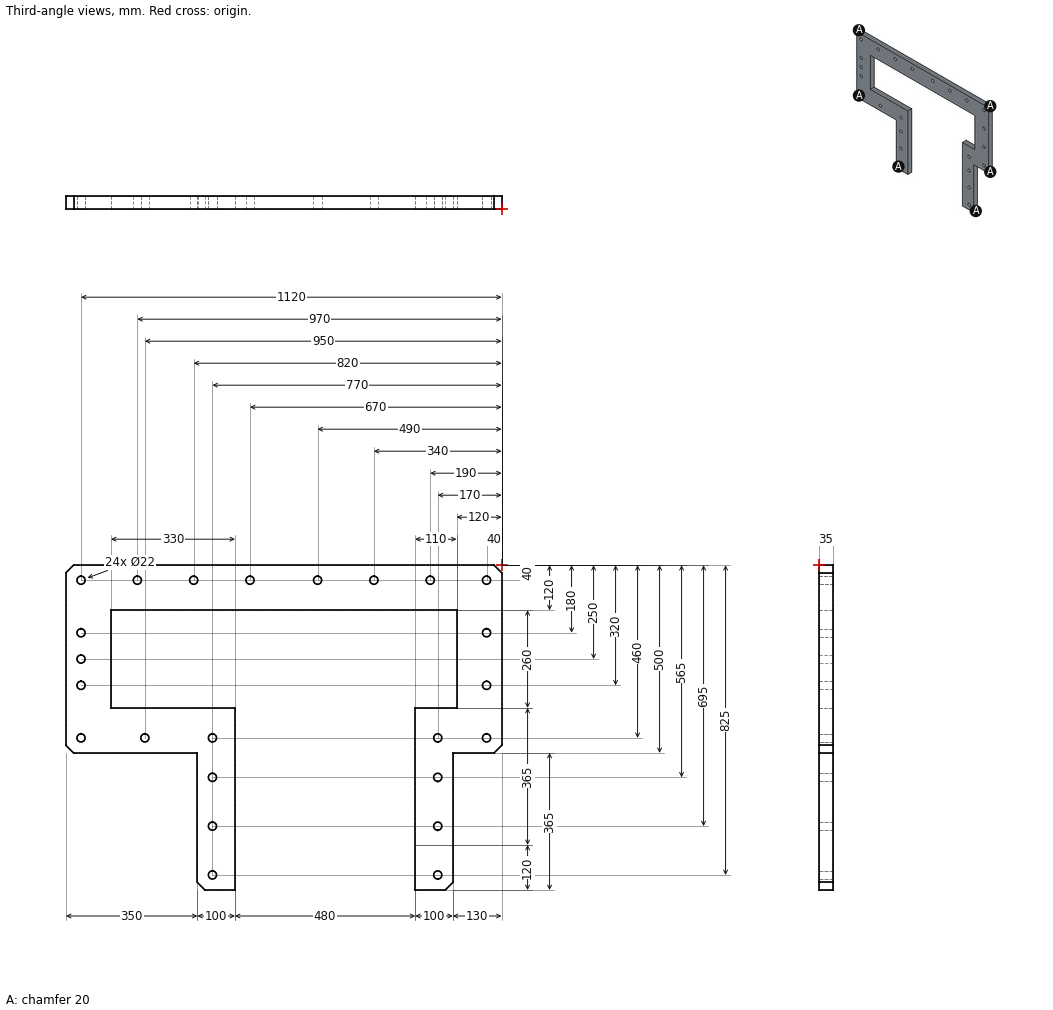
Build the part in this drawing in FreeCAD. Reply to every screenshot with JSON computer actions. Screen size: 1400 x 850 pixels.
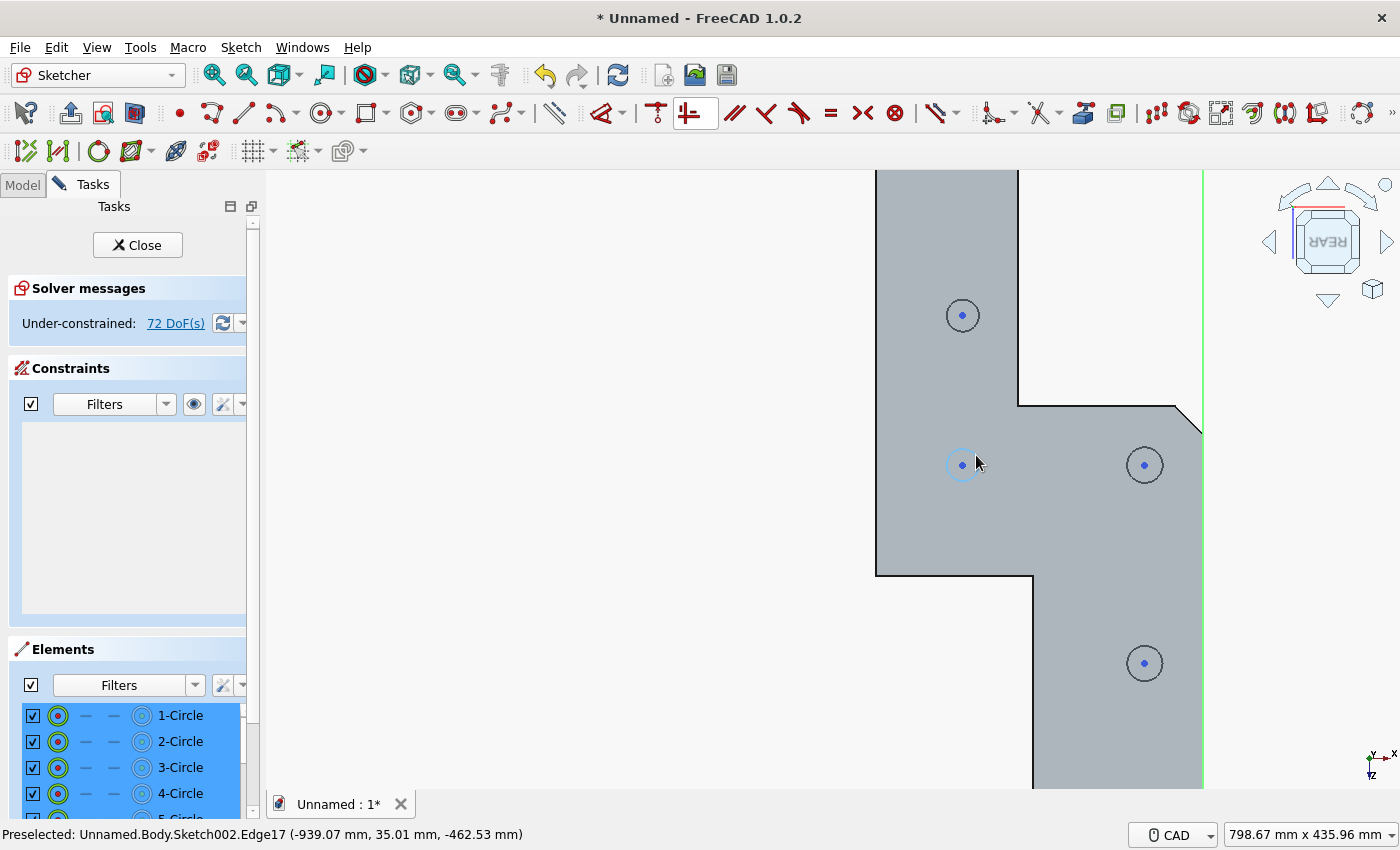
{"action": "left_click", "coordinate": [974, 454]}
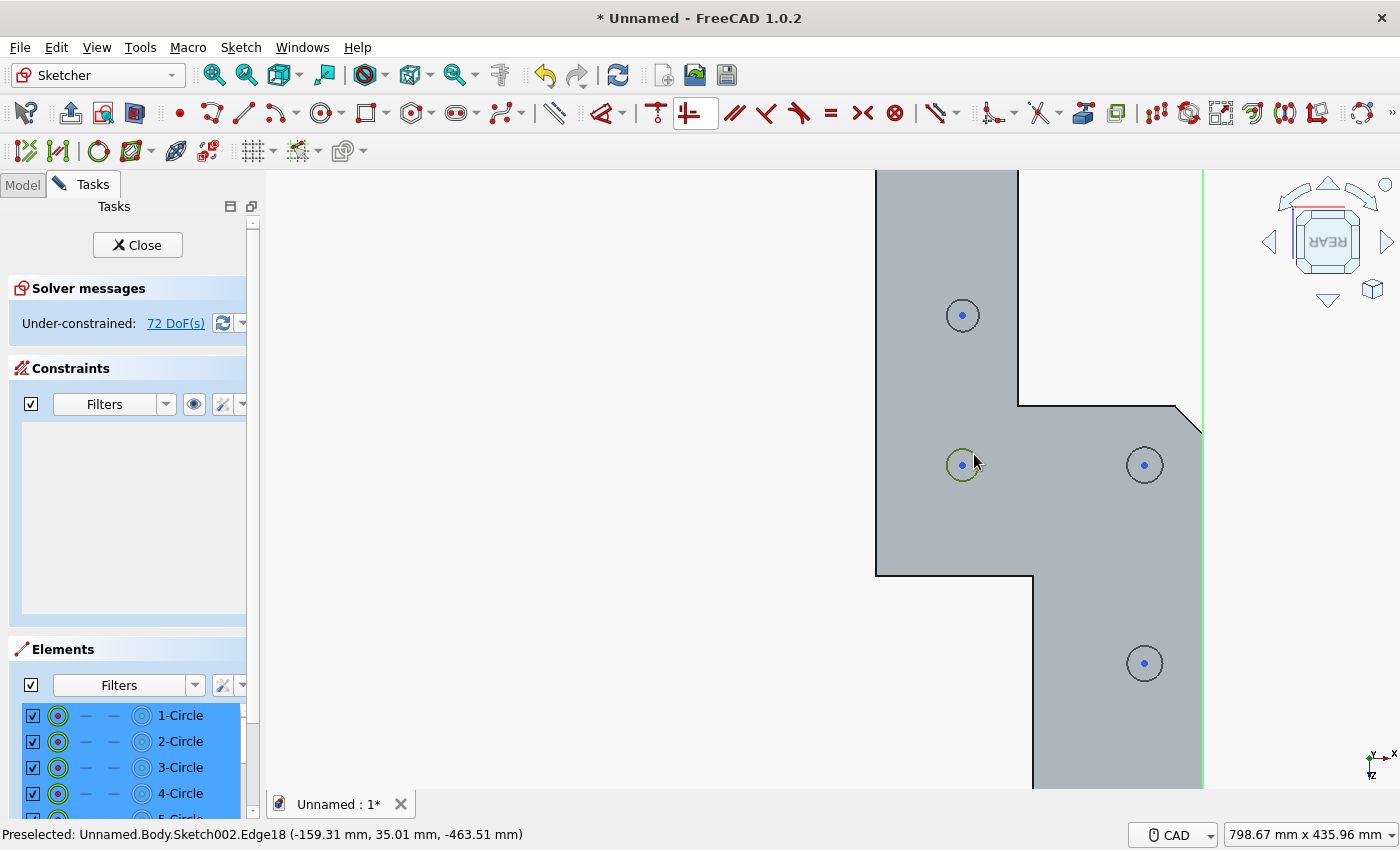
{"action": "left_click", "coordinate": [974, 304]}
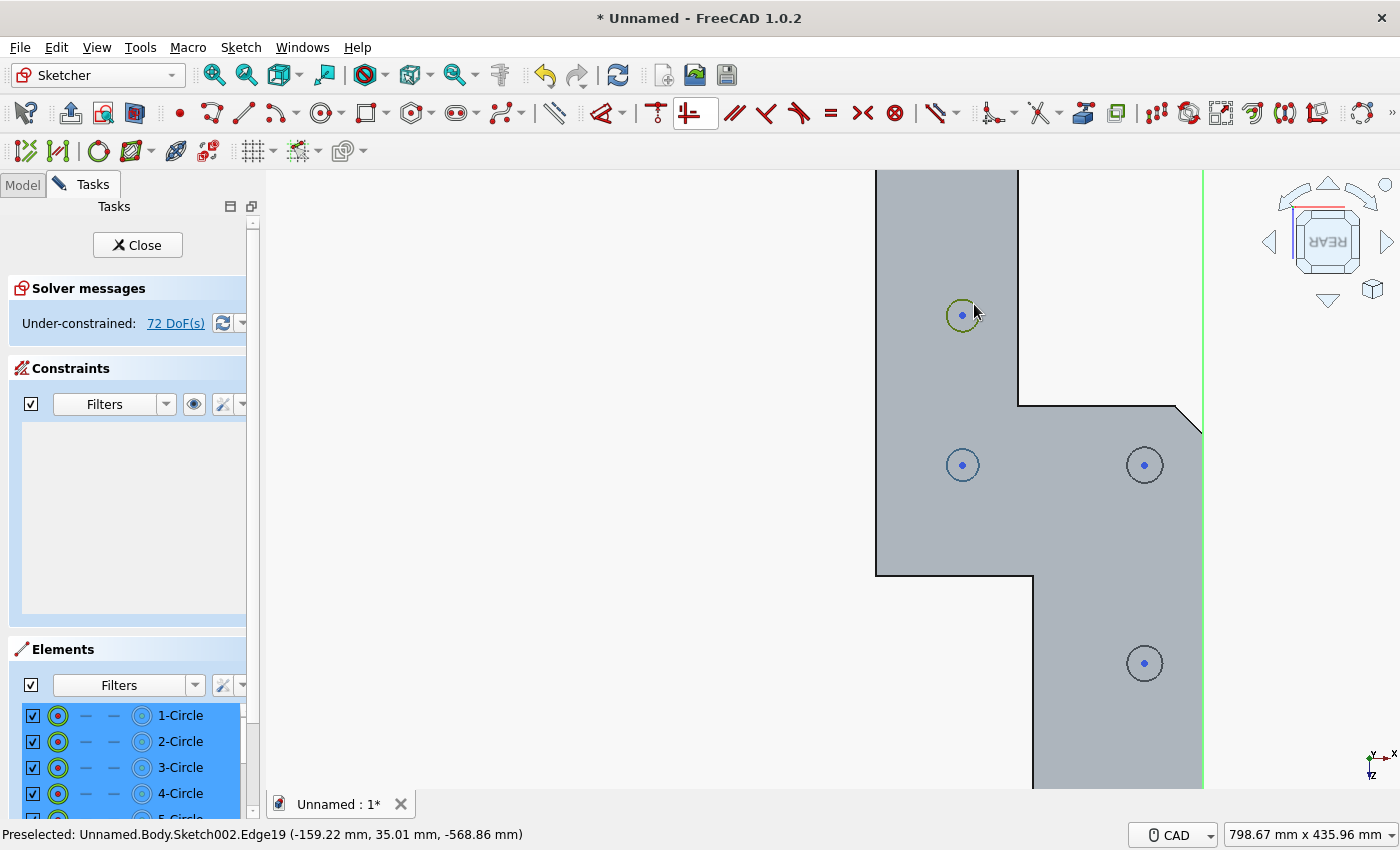
{"action": "scroll", "coordinate": [977, 455], "scroll_direction": "down", "scroll_amount": 5}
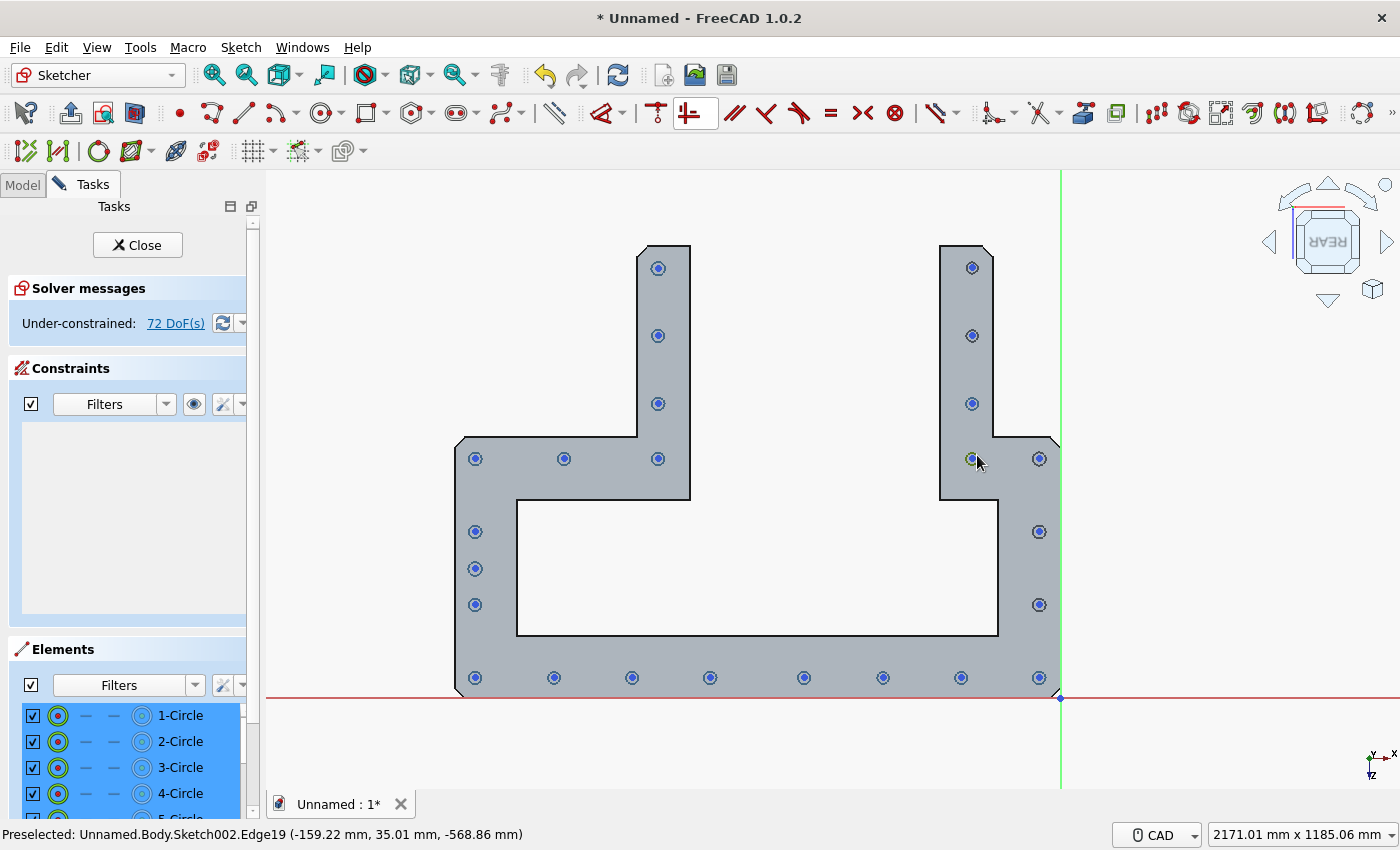
{"action": "scroll", "coordinate": [976, 332], "scroll_direction": "up", "scroll_amount": 5}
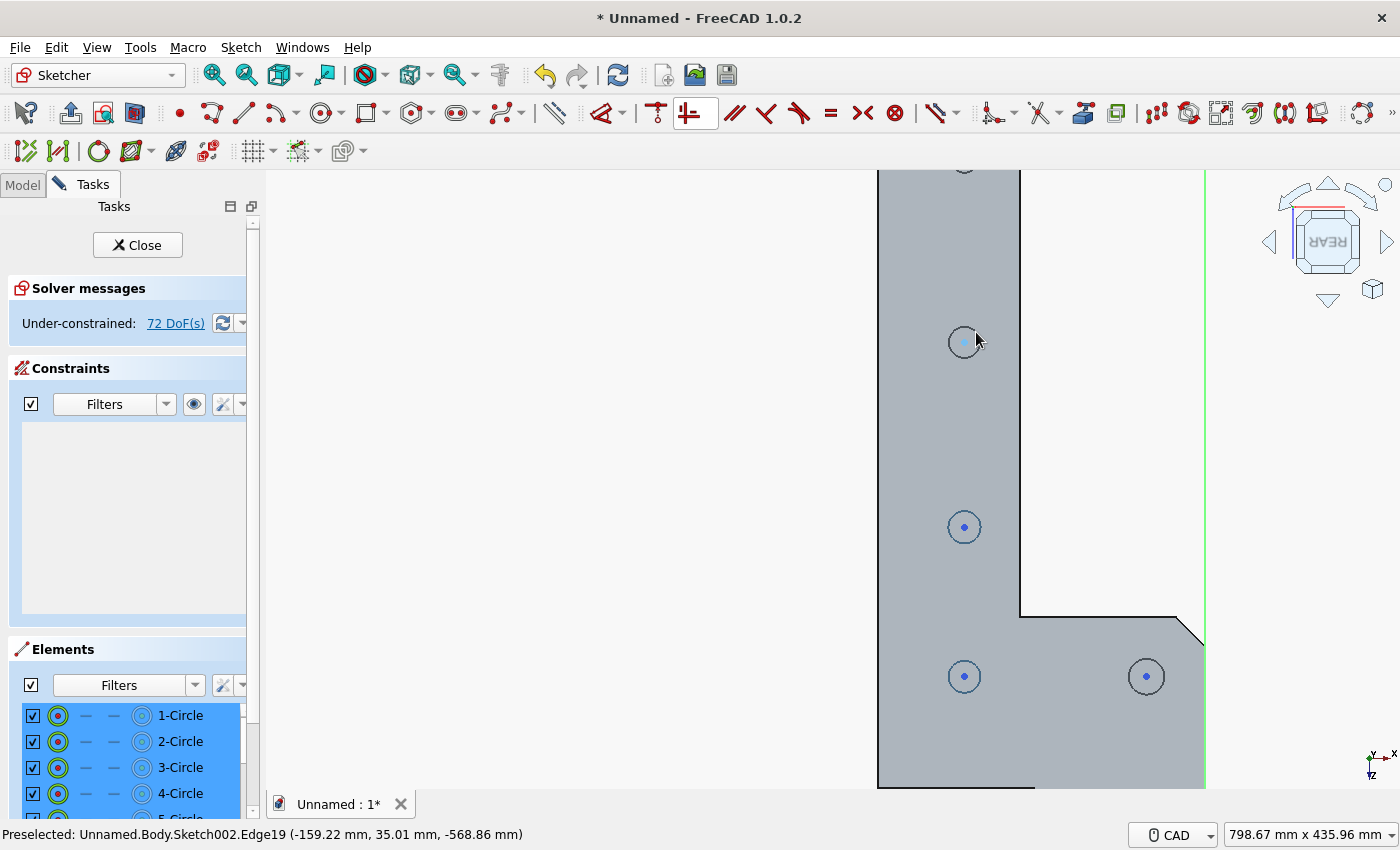
{"action": "left_click", "coordinate": [975, 331]}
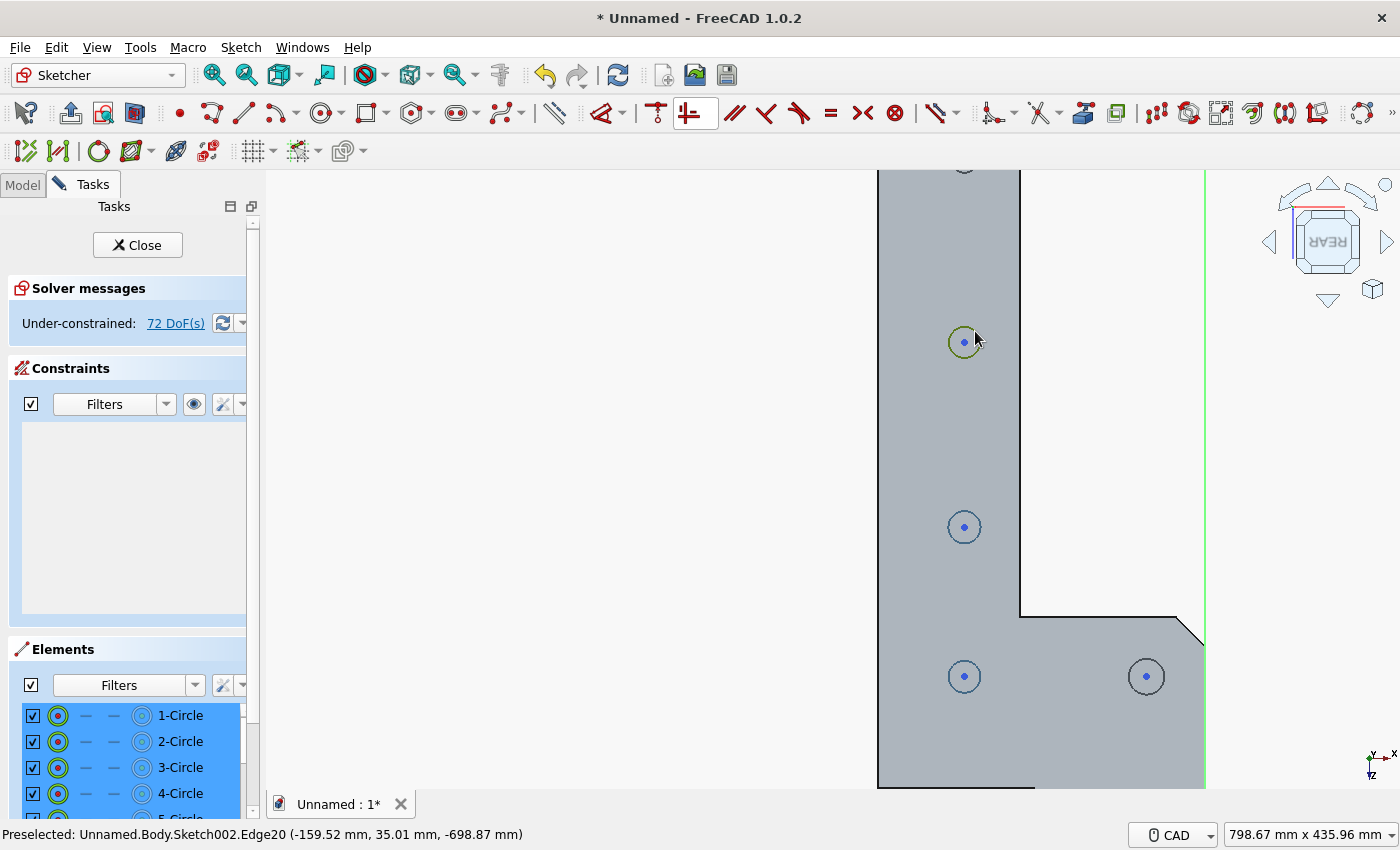
{"action": "scroll", "coordinate": [976, 332], "scroll_direction": "down", "scroll_amount": 5}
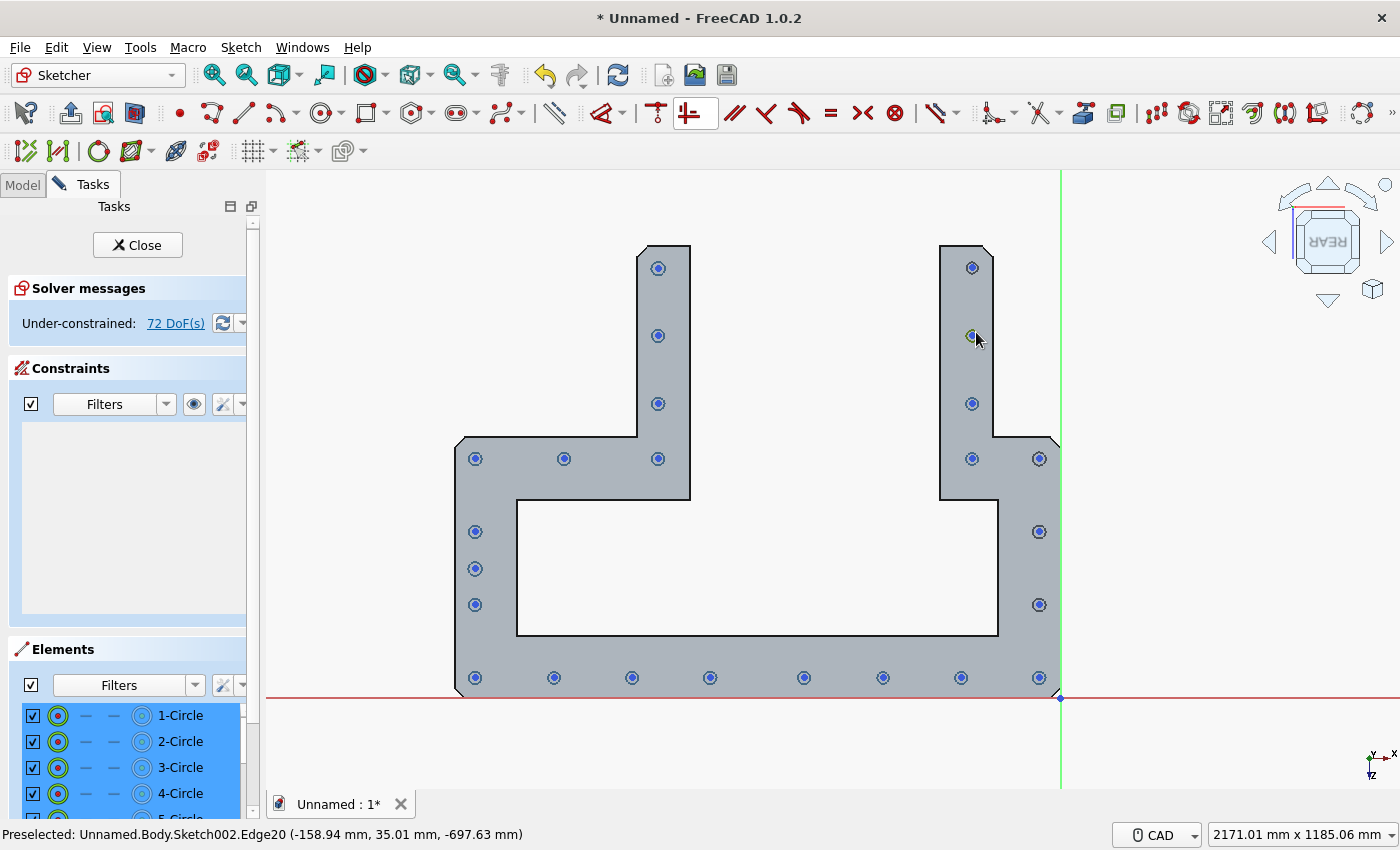
{"action": "scroll", "coordinate": [976, 264], "scroll_direction": "up", "scroll_amount": 5}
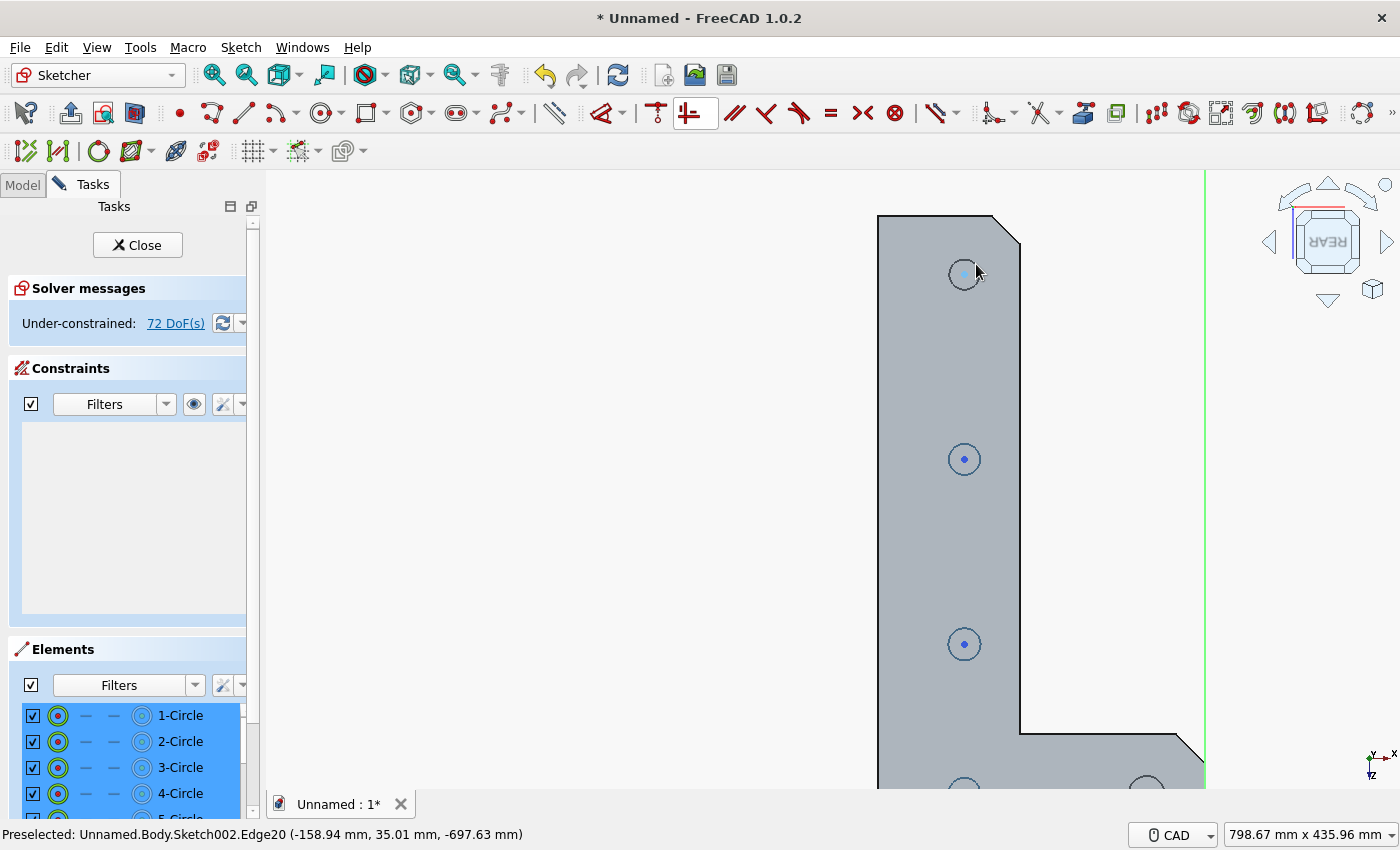
{"action": "left_click", "coordinate": [975, 264]}